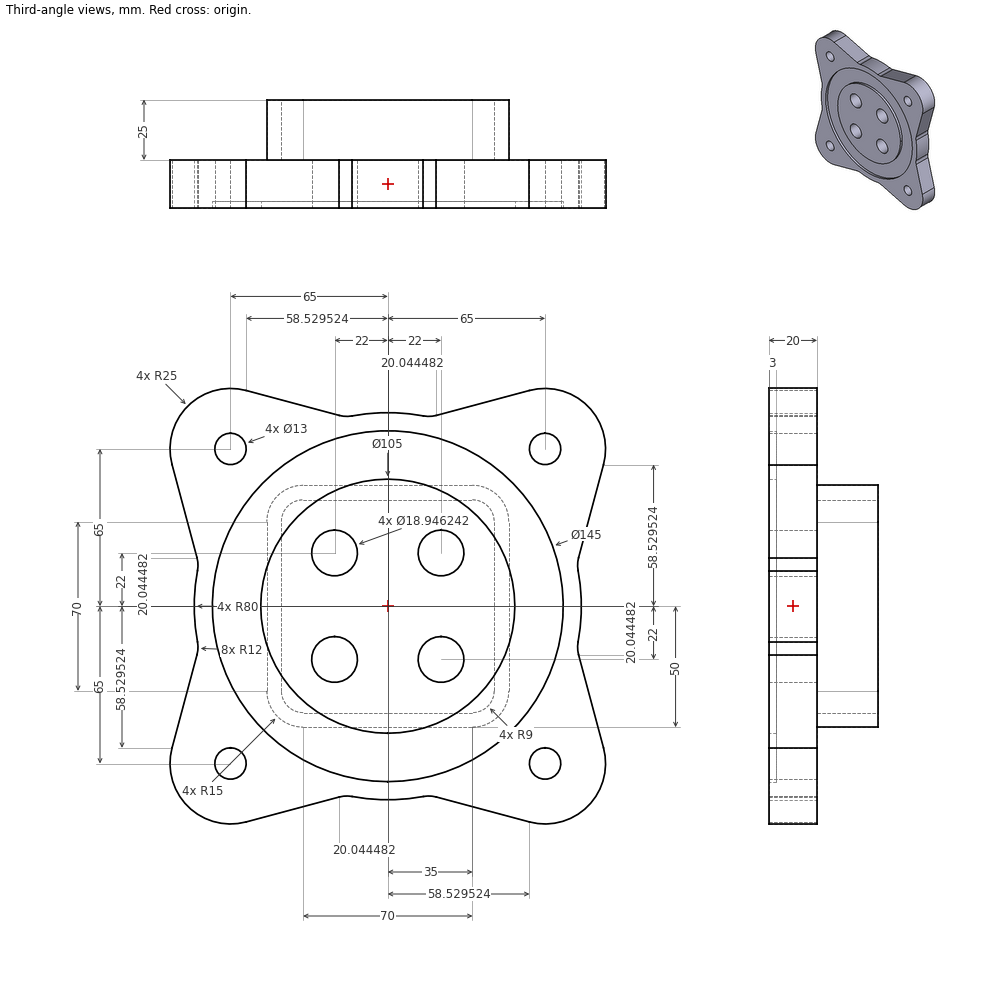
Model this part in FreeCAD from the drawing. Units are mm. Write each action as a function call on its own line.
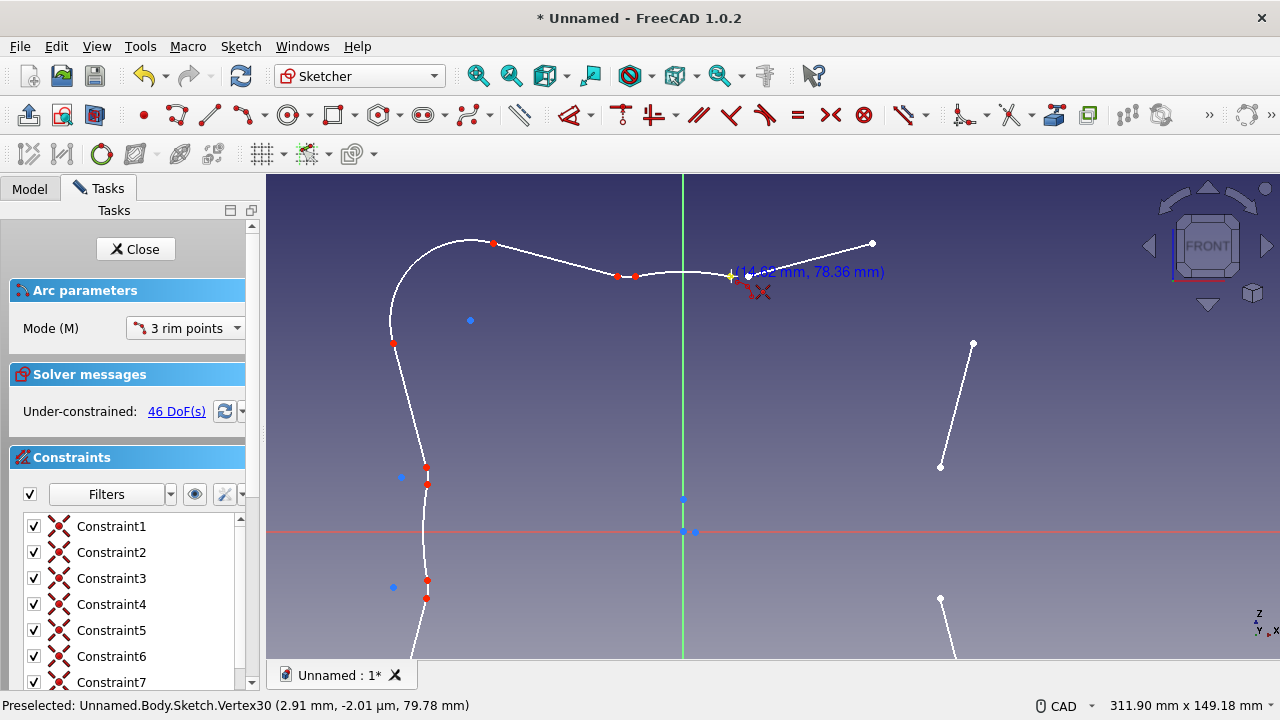
click(731, 277)
click(749, 276)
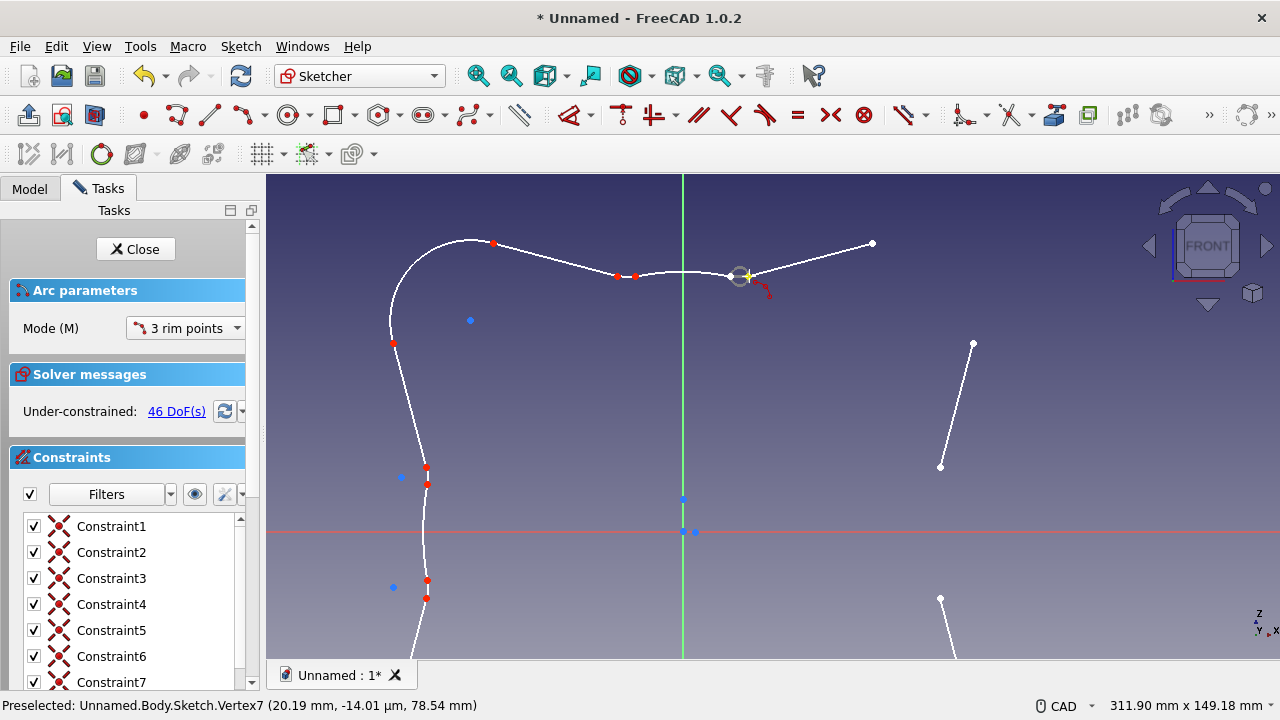
scroll(740, 277, up, 14)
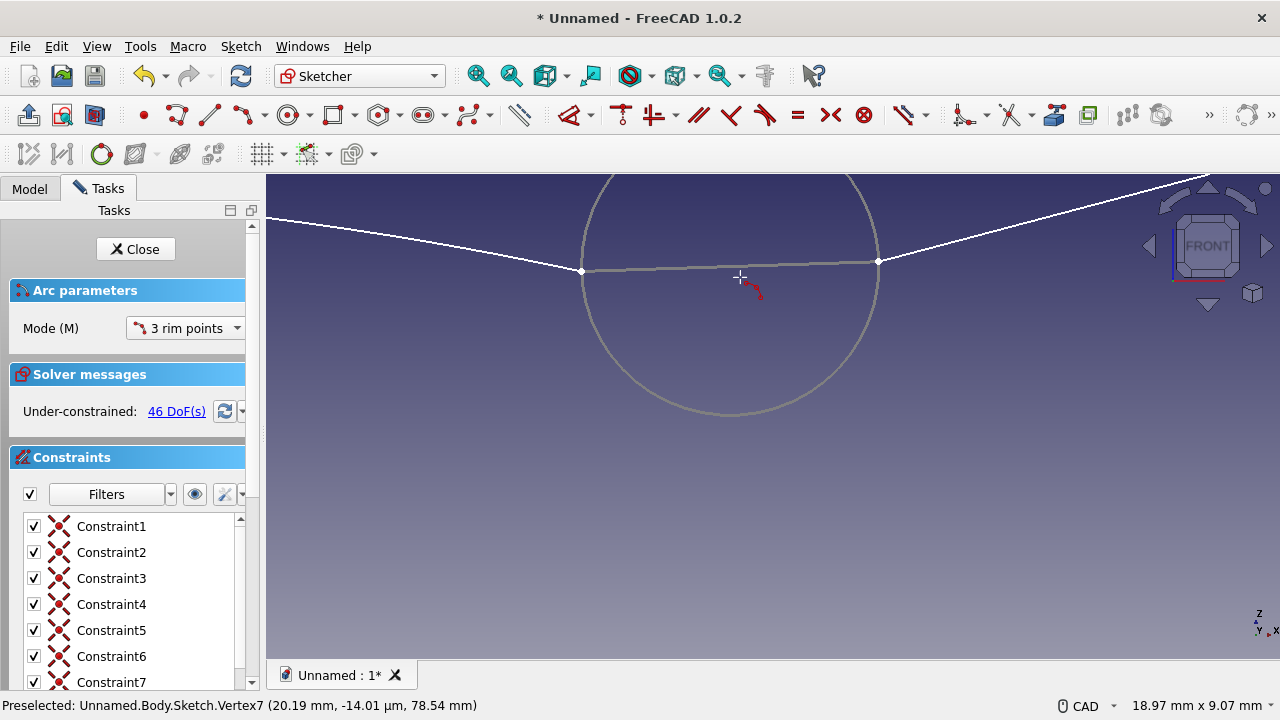
click(730, 267)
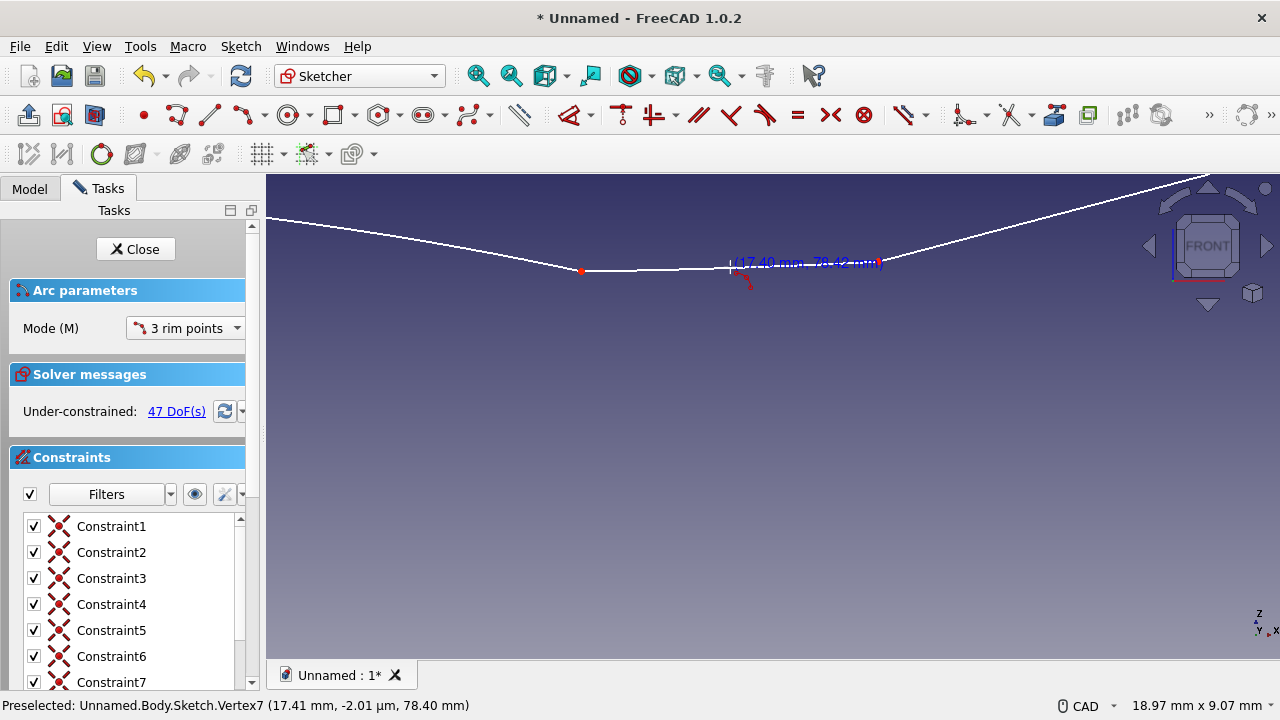
scroll(736, 277, down, 17)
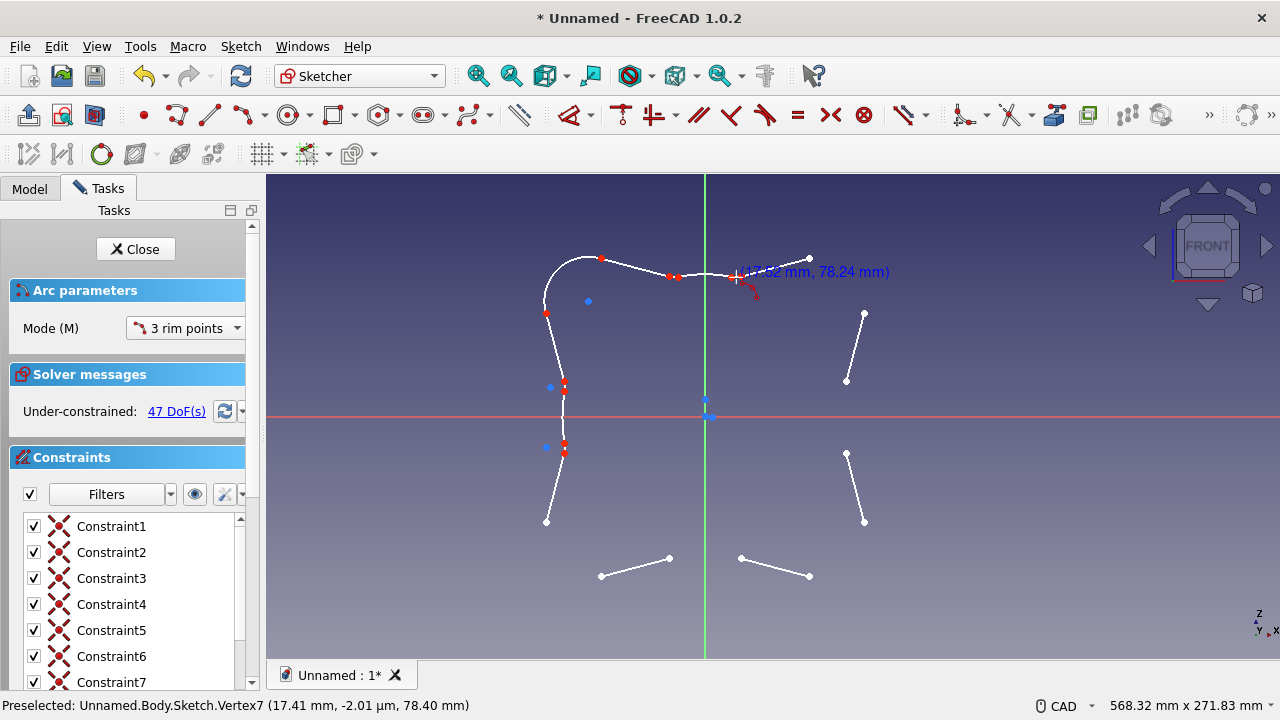
click(809, 259)
click(864, 314)
click(853, 269)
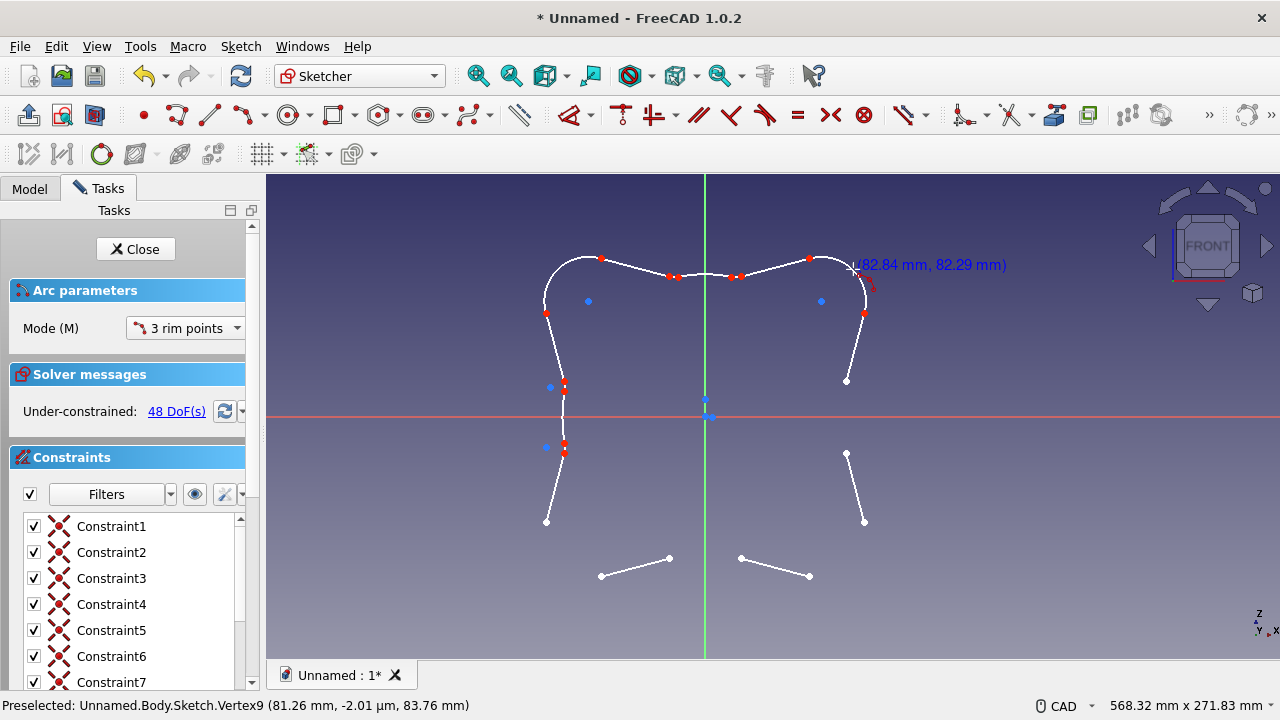
click(846, 382)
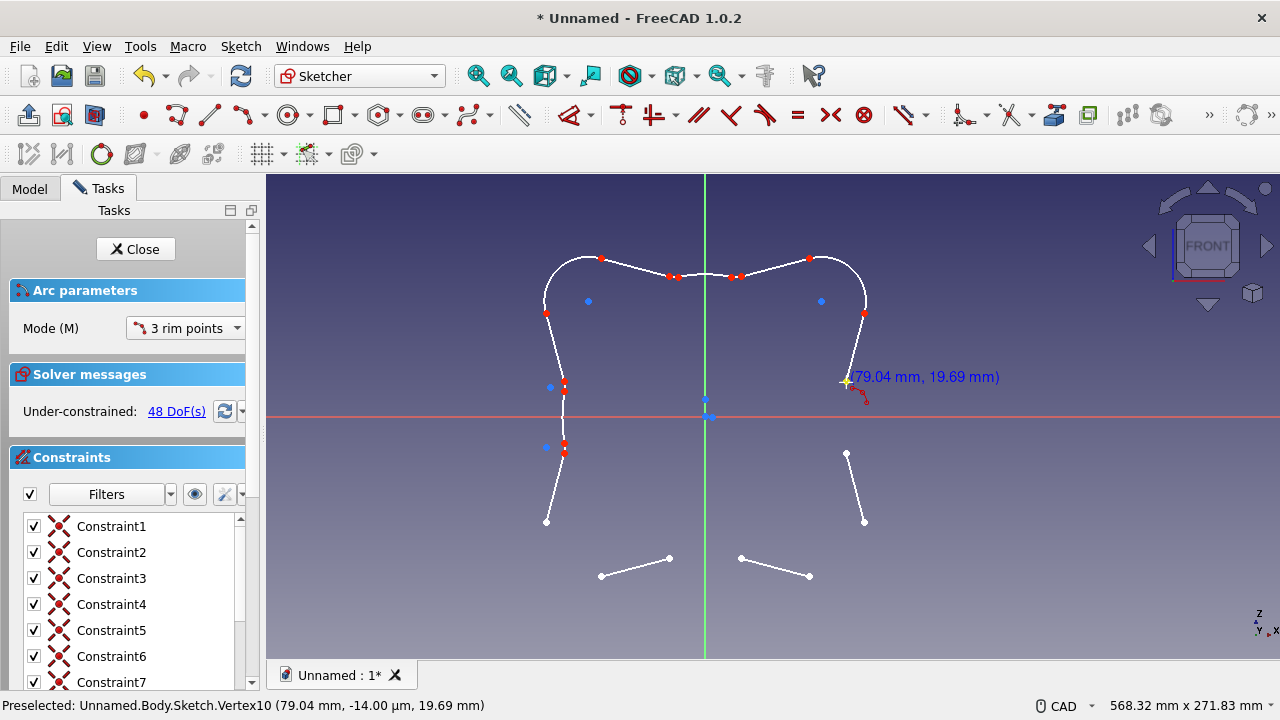
scroll(845, 391, up, 3)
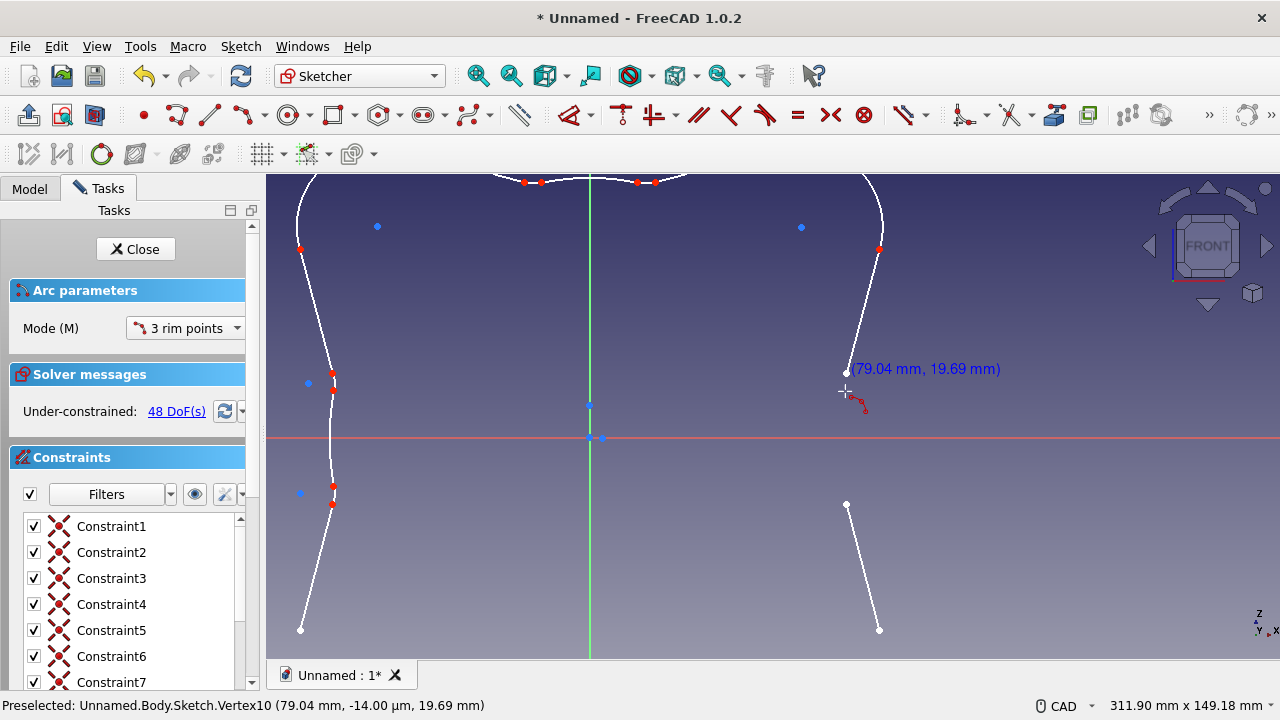
click(845, 390)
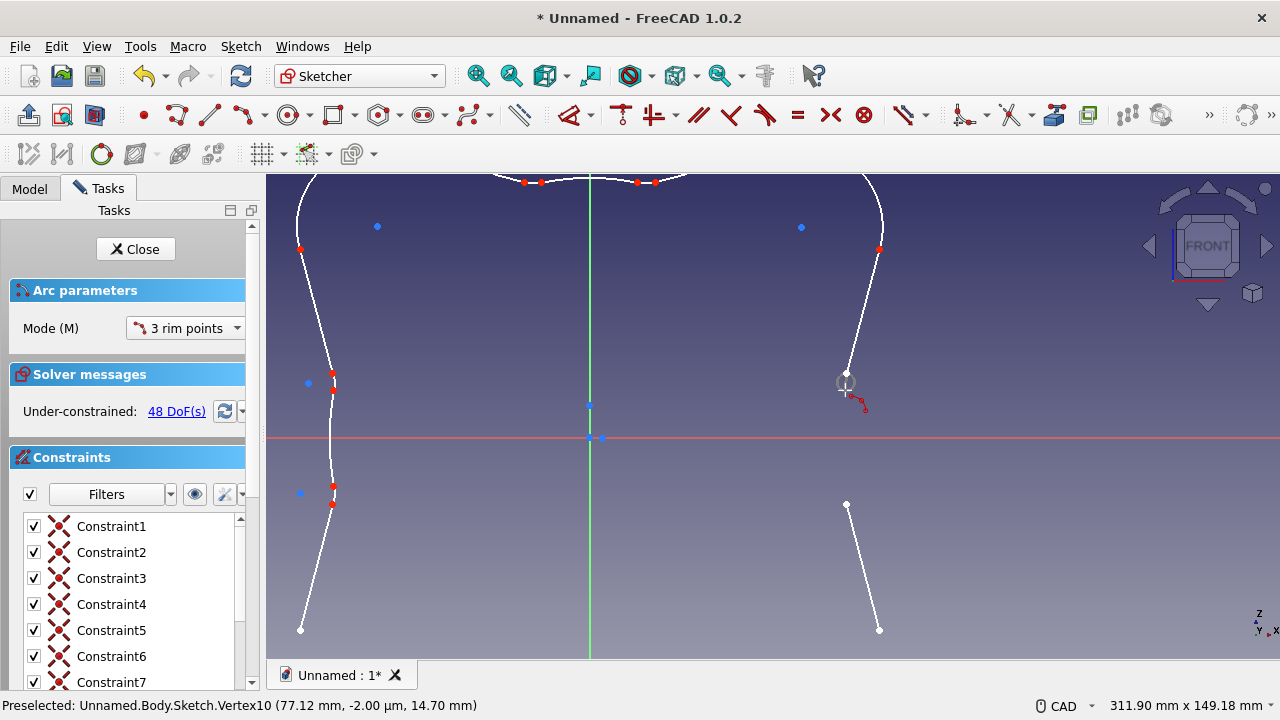
scroll(845, 381, up, 14)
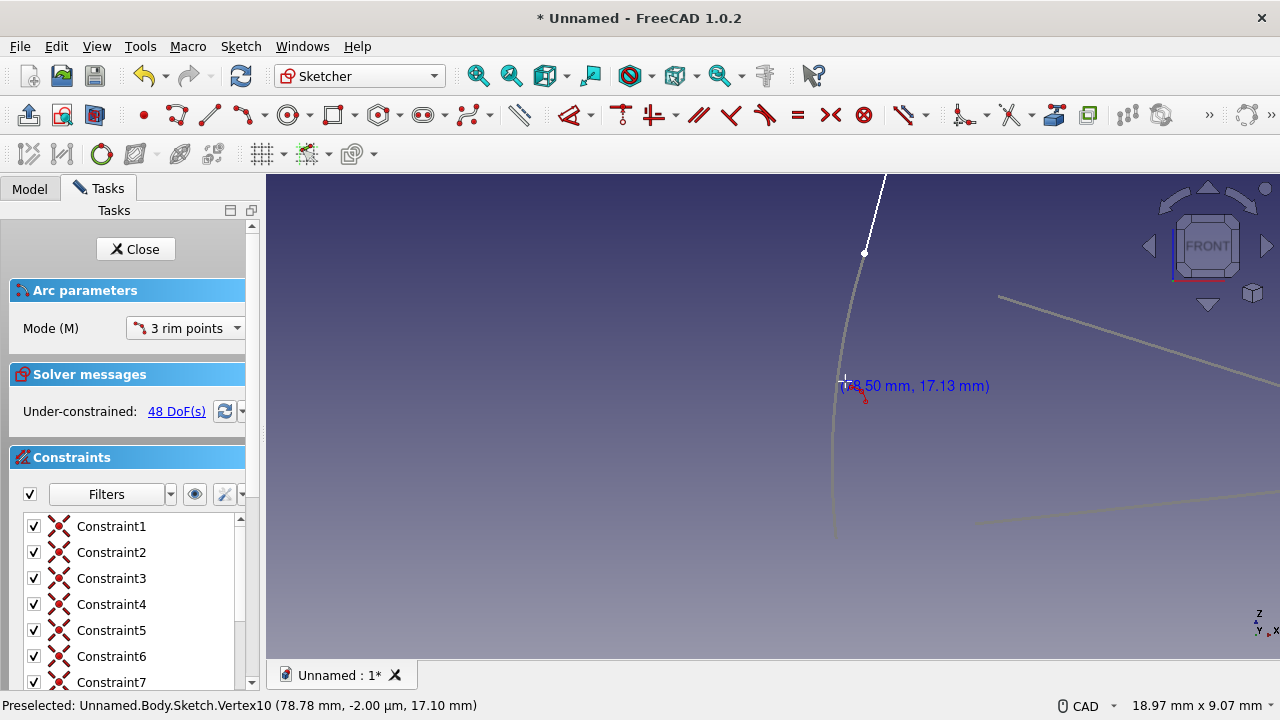
click(833, 377)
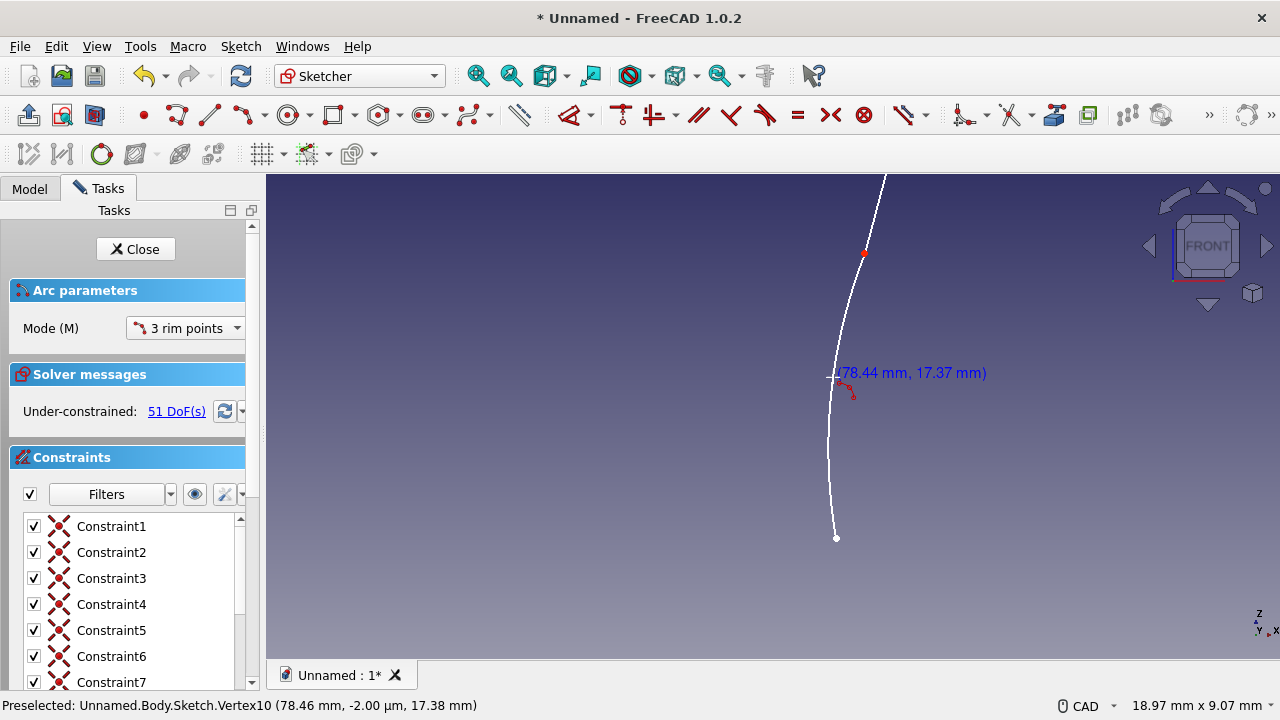
scroll(845, 386, down, 17)